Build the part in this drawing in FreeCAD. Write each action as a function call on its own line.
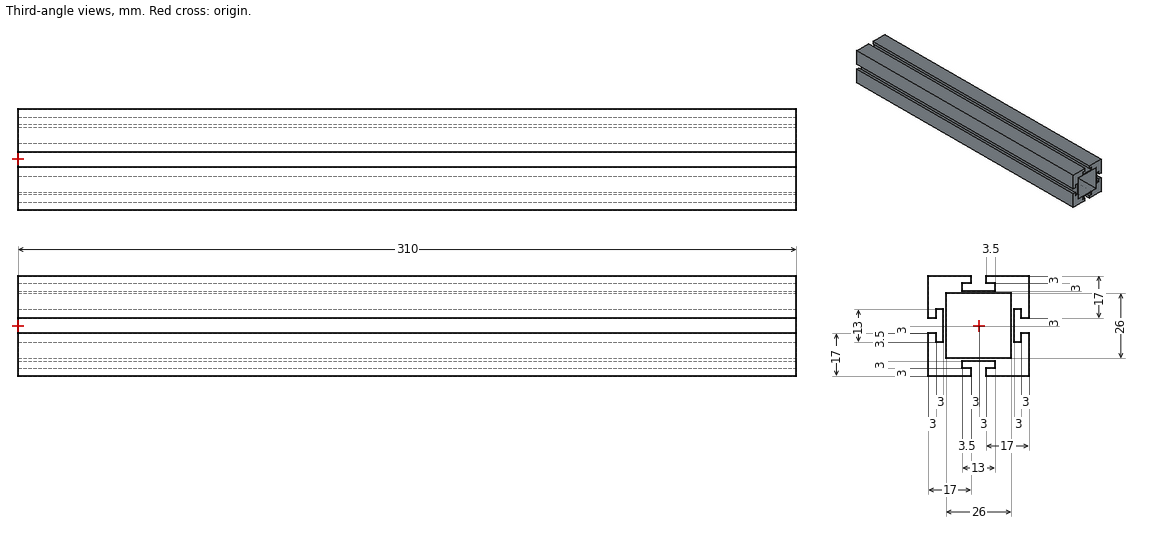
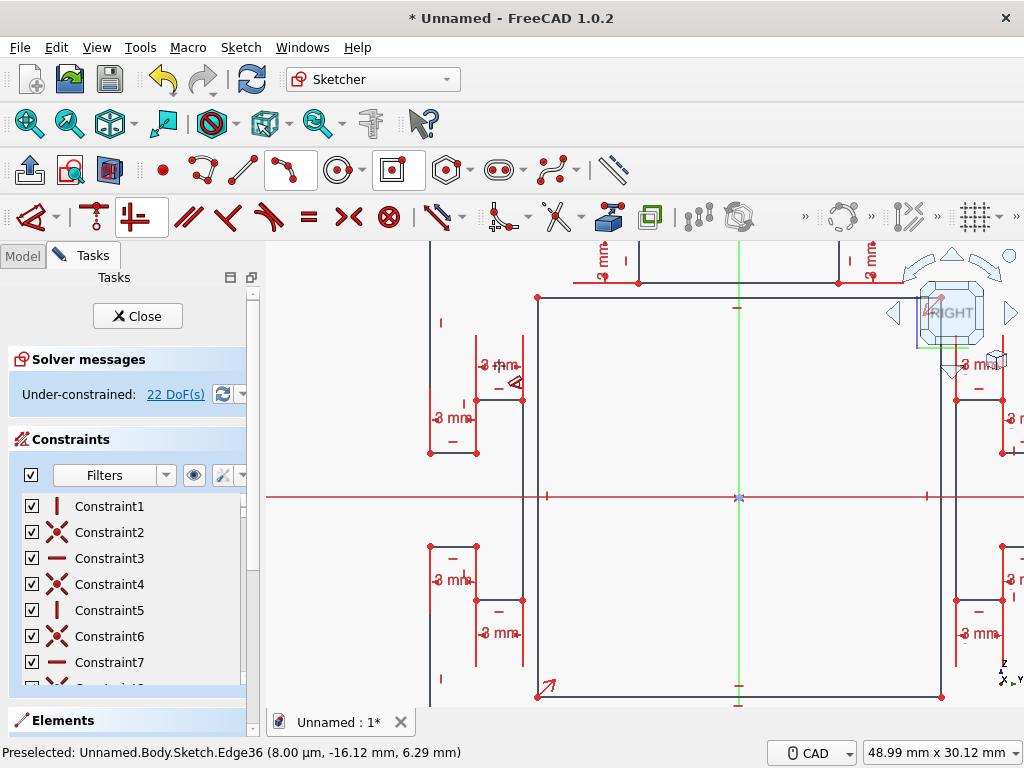
click(523, 460)
click(557, 454)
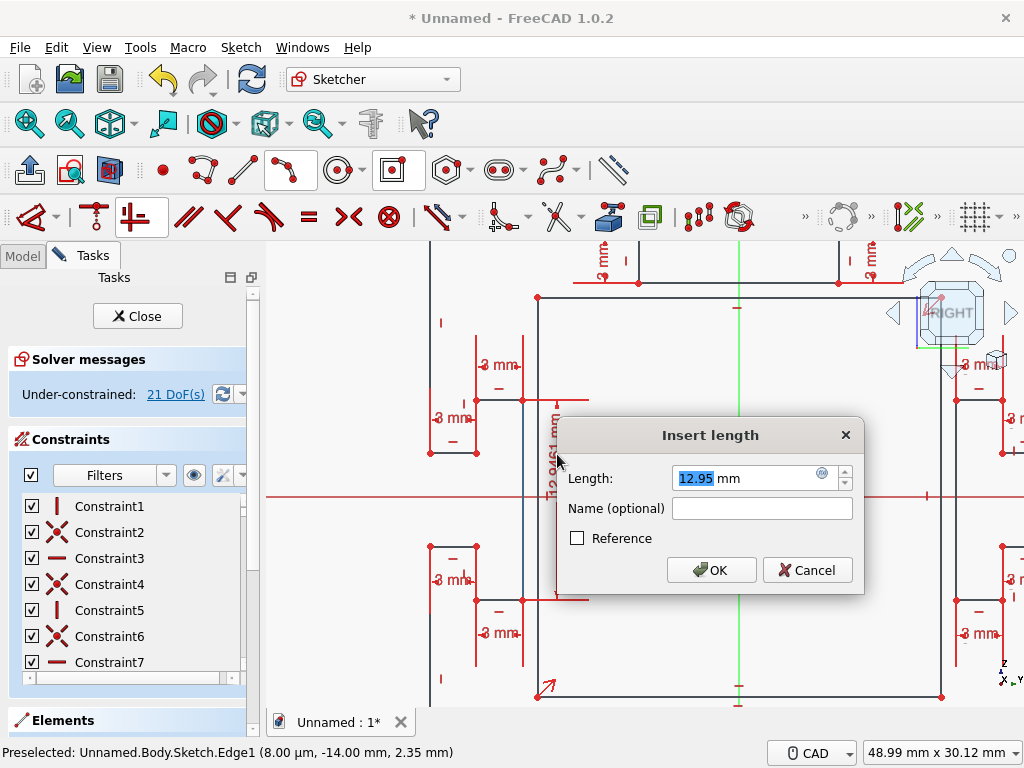
text(13)
key(Return)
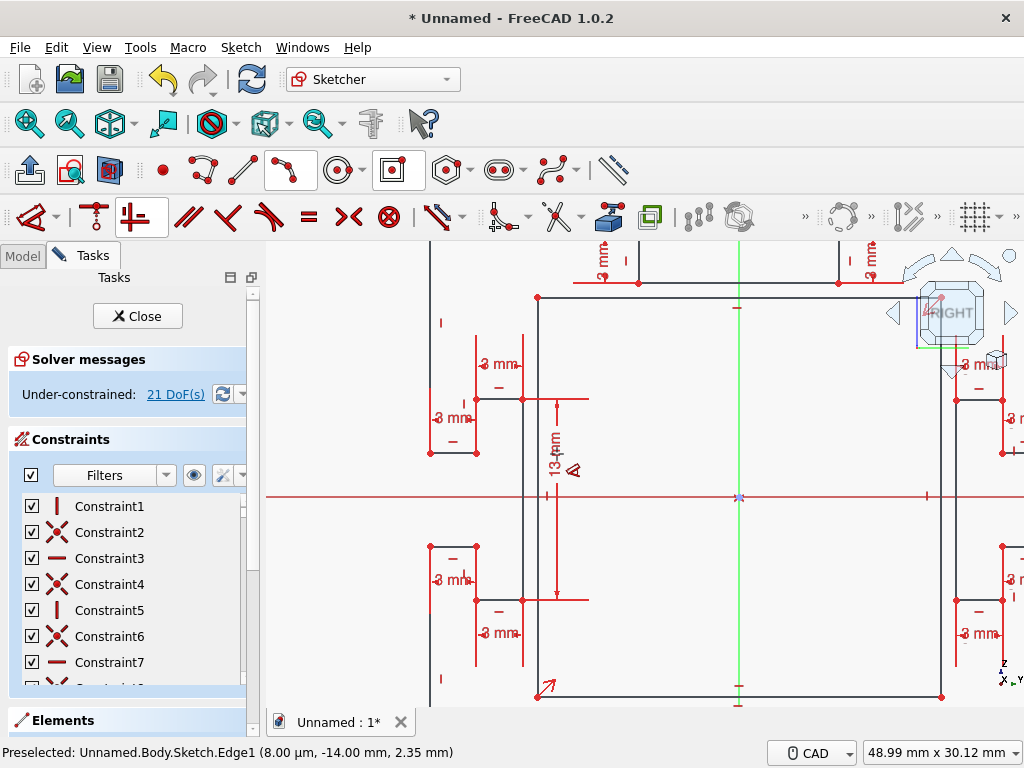
click(430, 626)
click(396, 613)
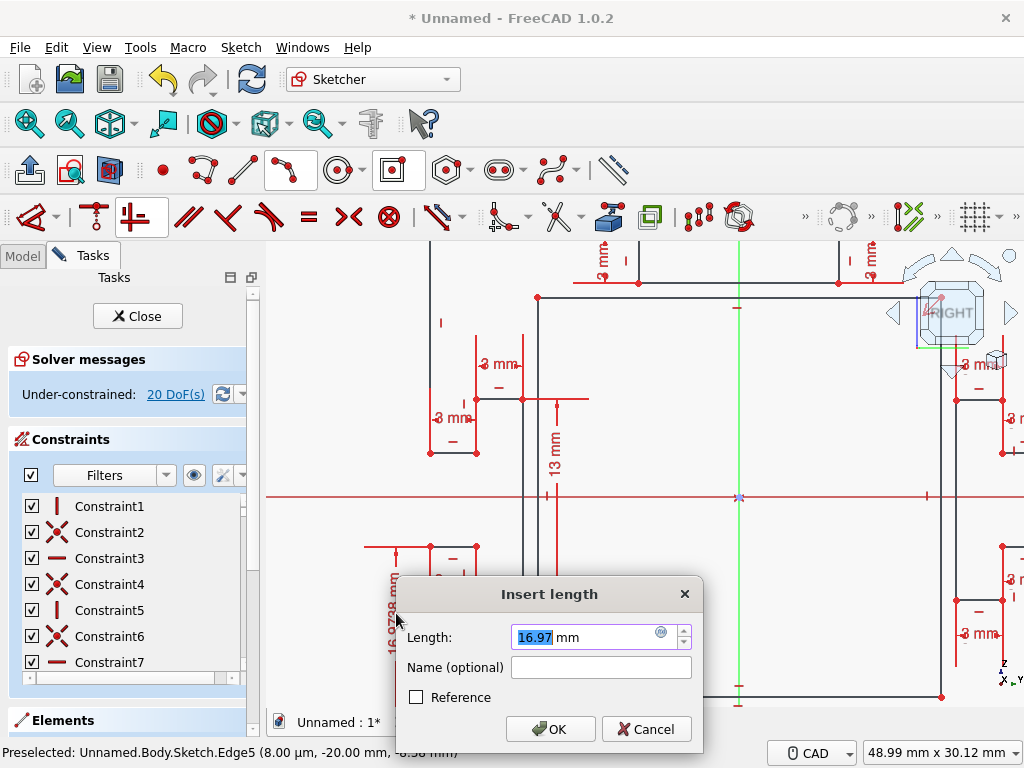
text(17)
key(Return)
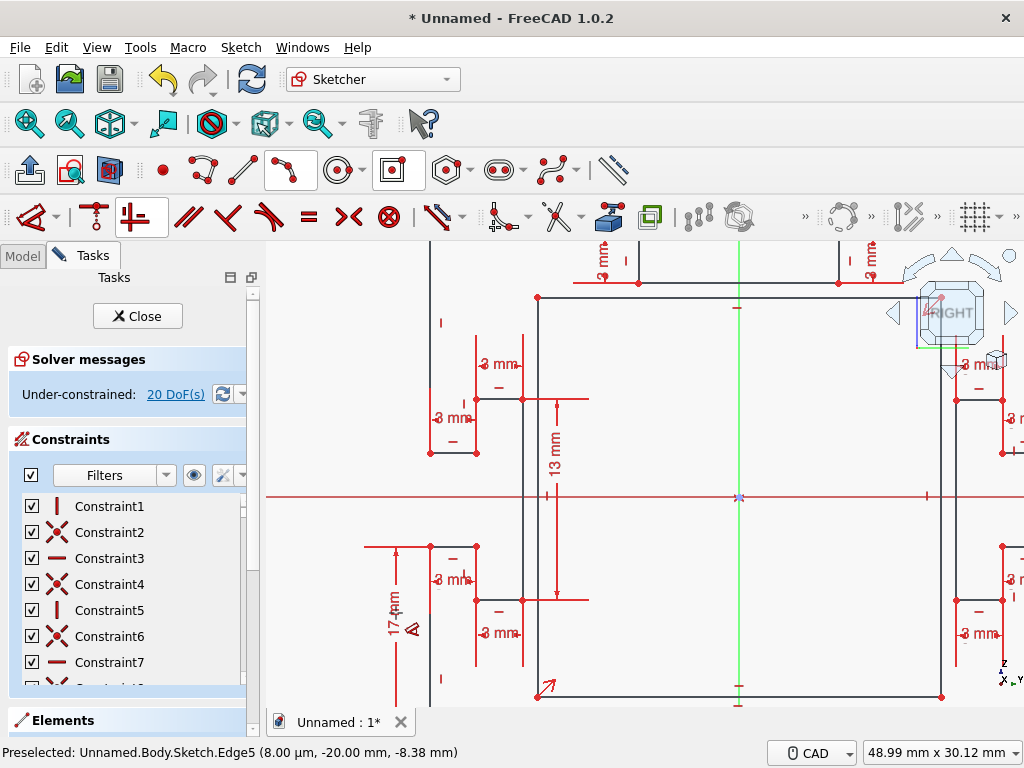
scroll(444, 455, down, 4)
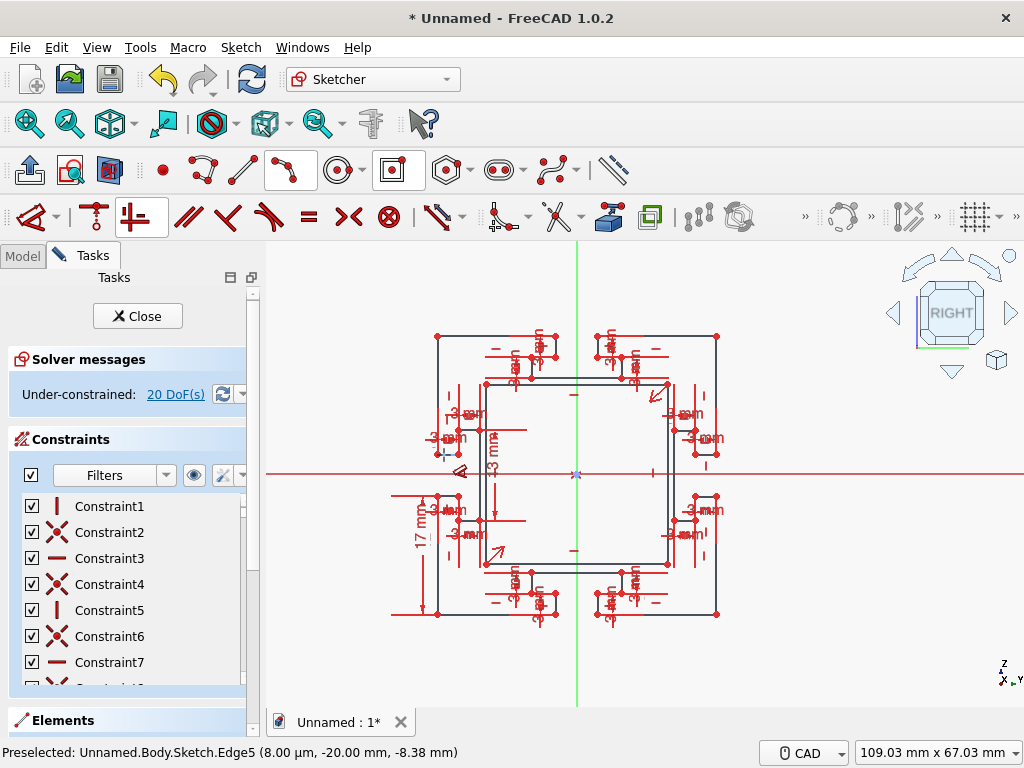
click(473, 615)
click(497, 649)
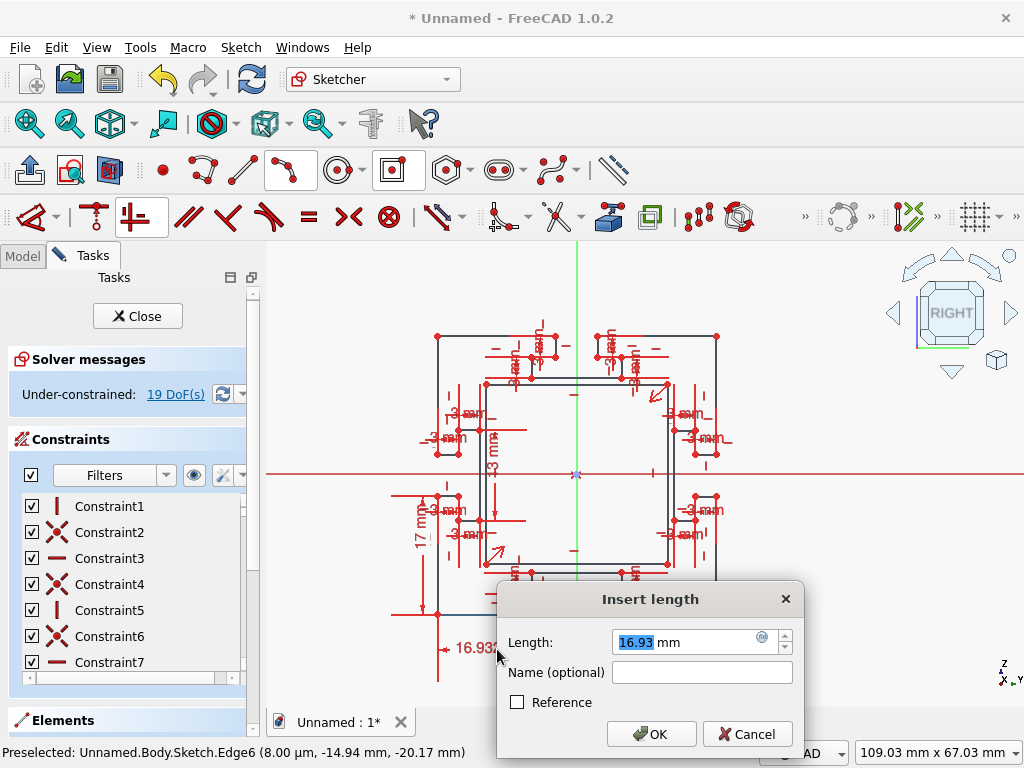
text(17)
key(Return)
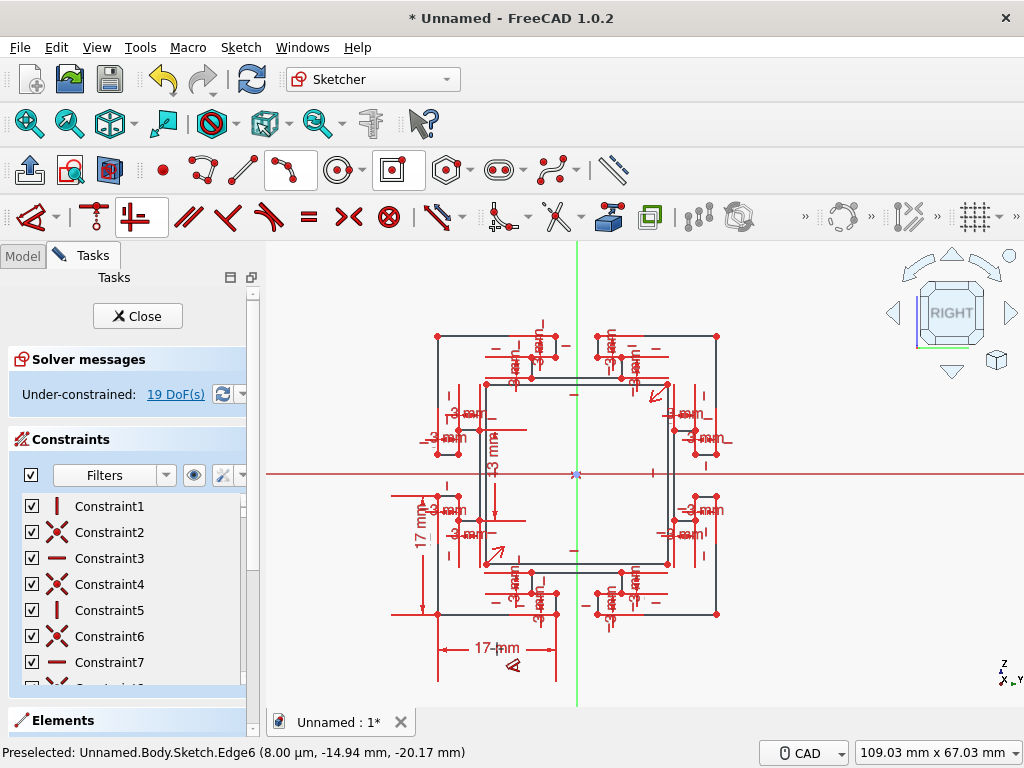
scroll(559, 573, up, 3)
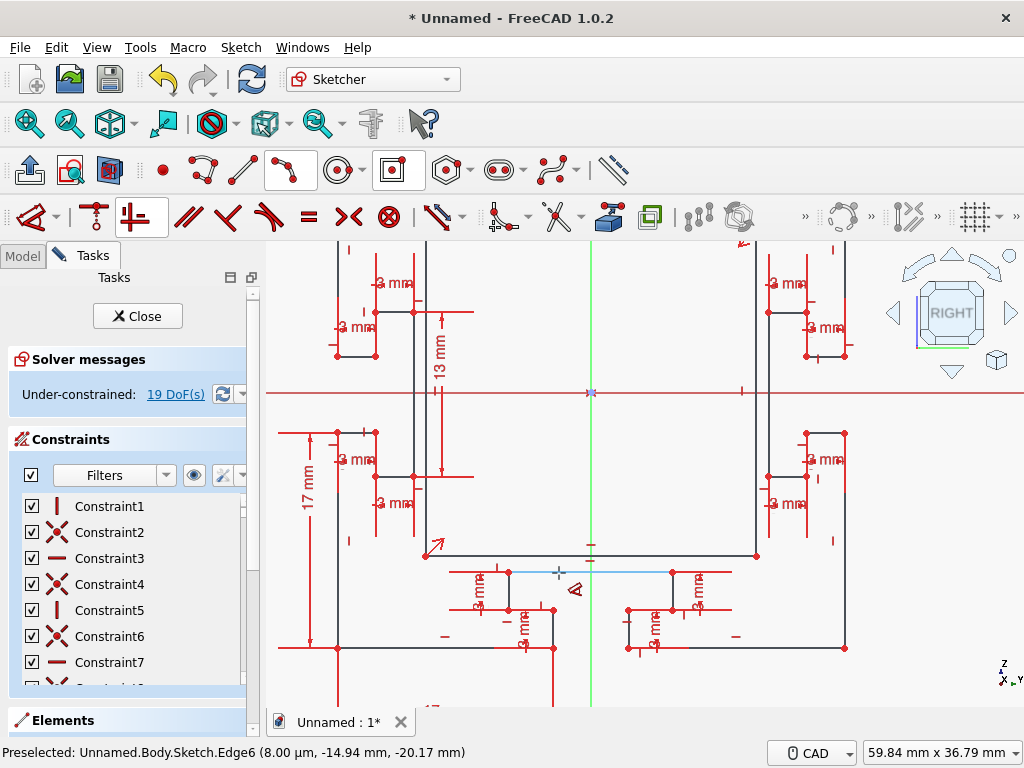
click(558, 572)
click(553, 538)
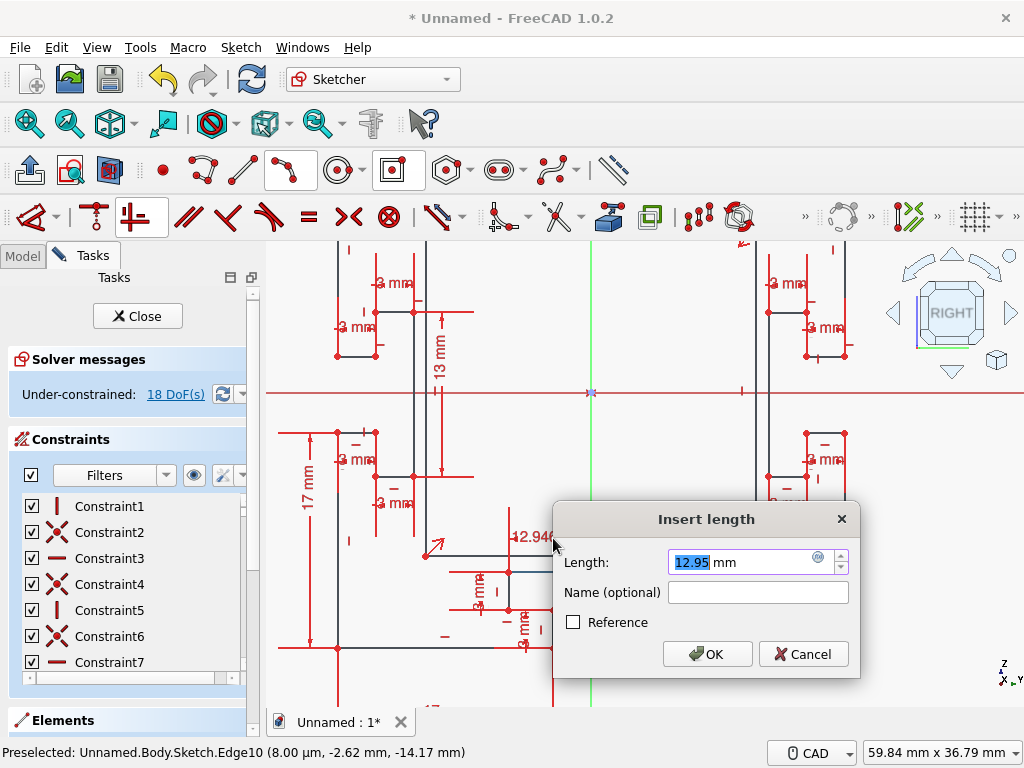
text(13)
key(Return)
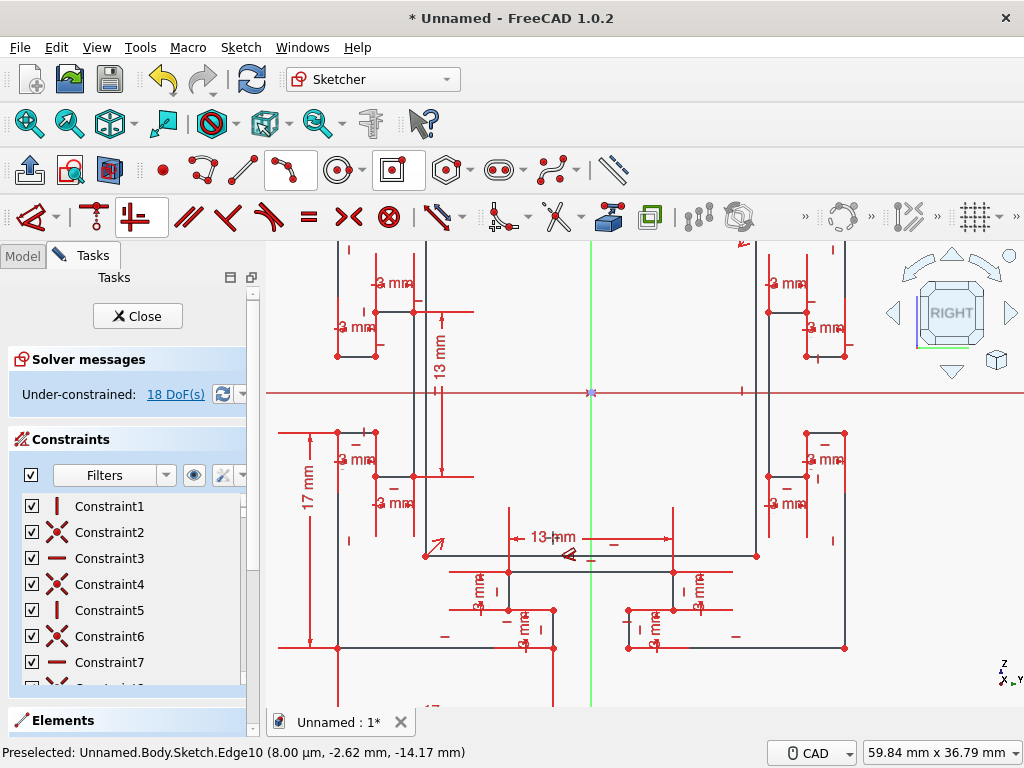
click(694, 648)
click(737, 614)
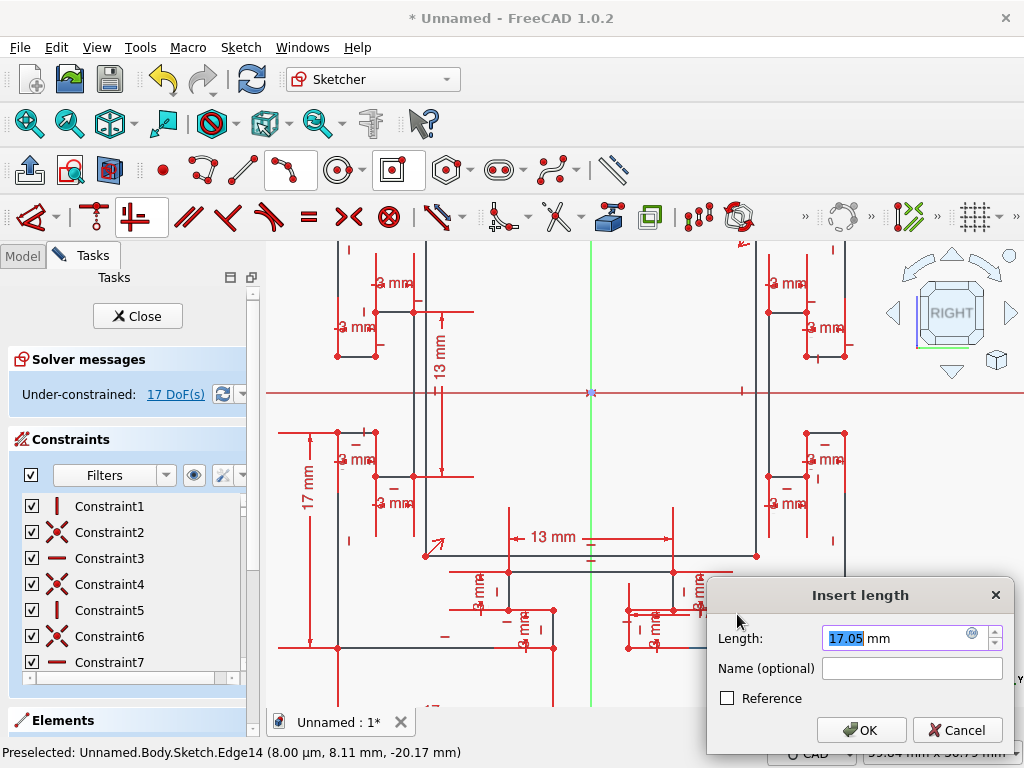
text(17)
key(Return)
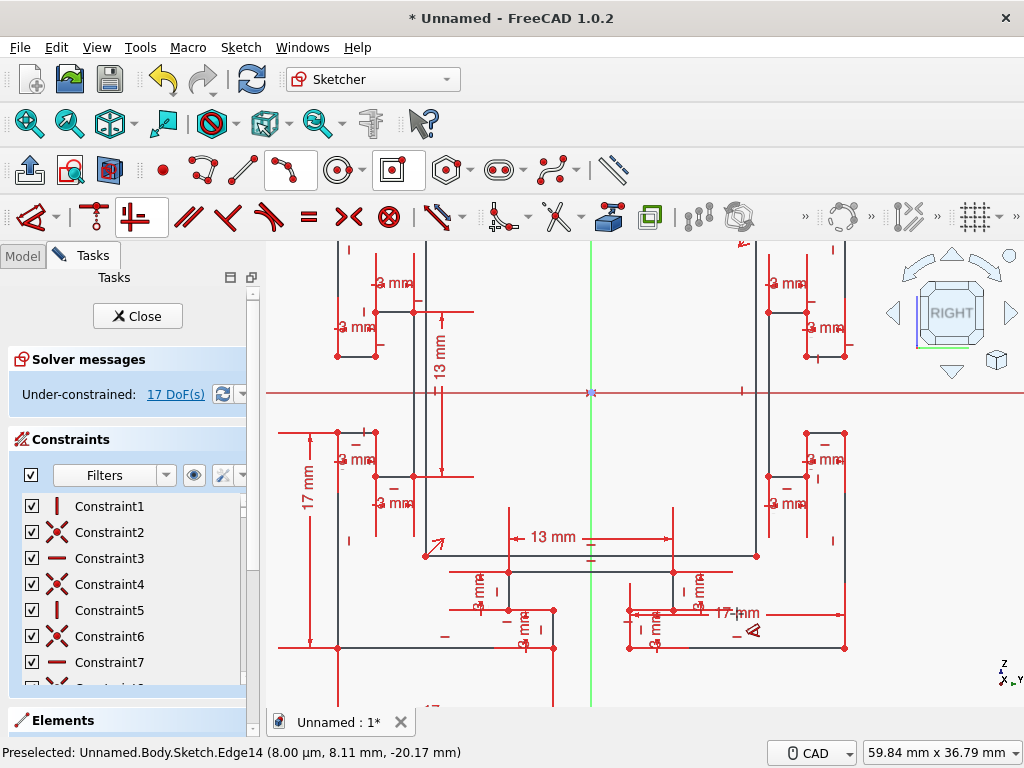
click(845, 584)
click(811, 541)